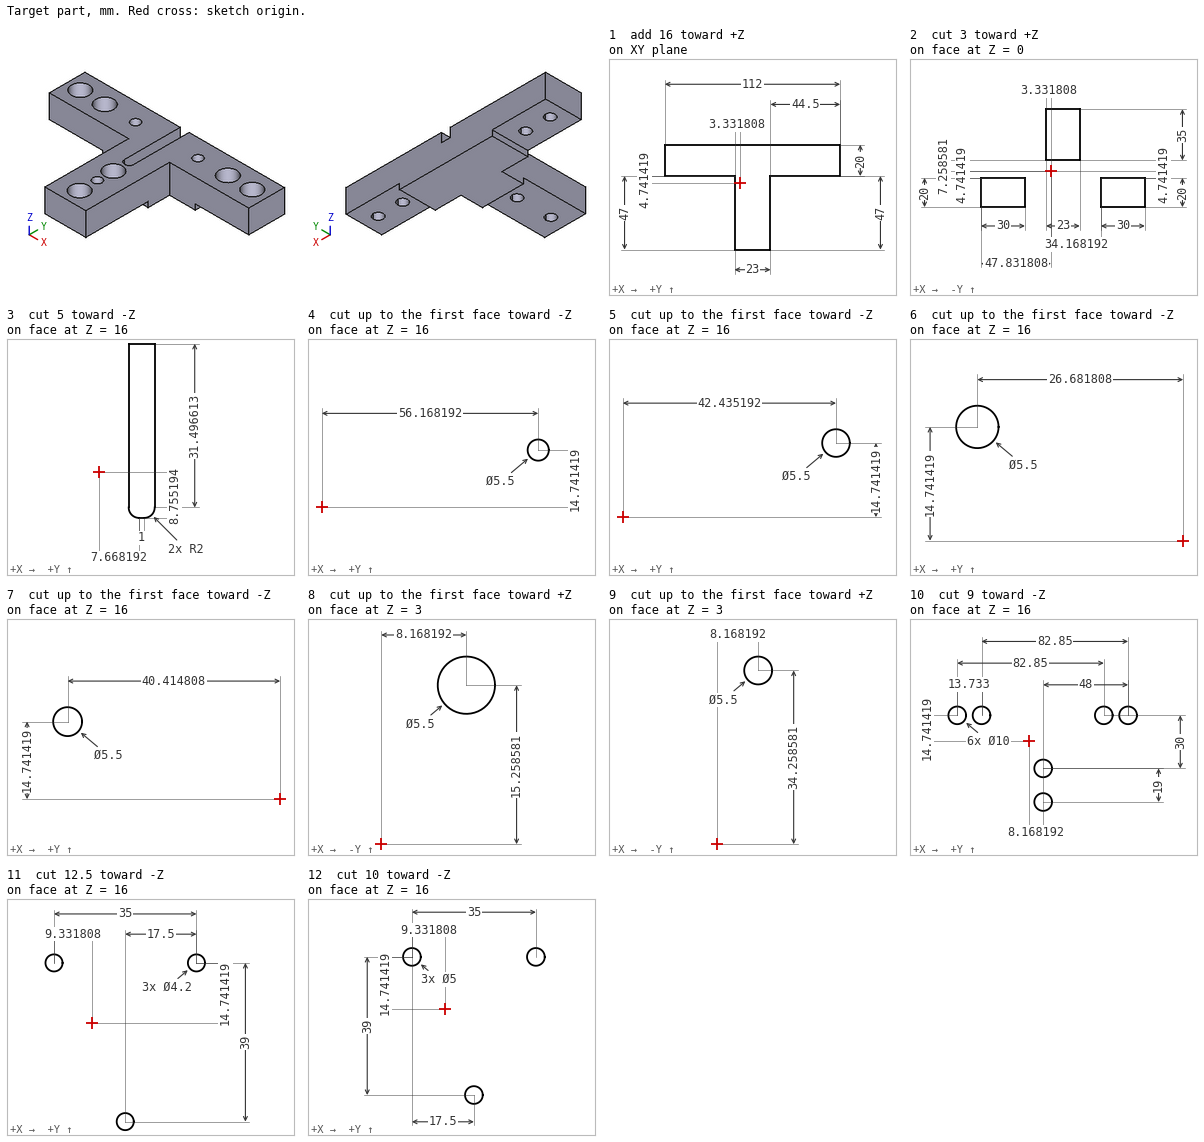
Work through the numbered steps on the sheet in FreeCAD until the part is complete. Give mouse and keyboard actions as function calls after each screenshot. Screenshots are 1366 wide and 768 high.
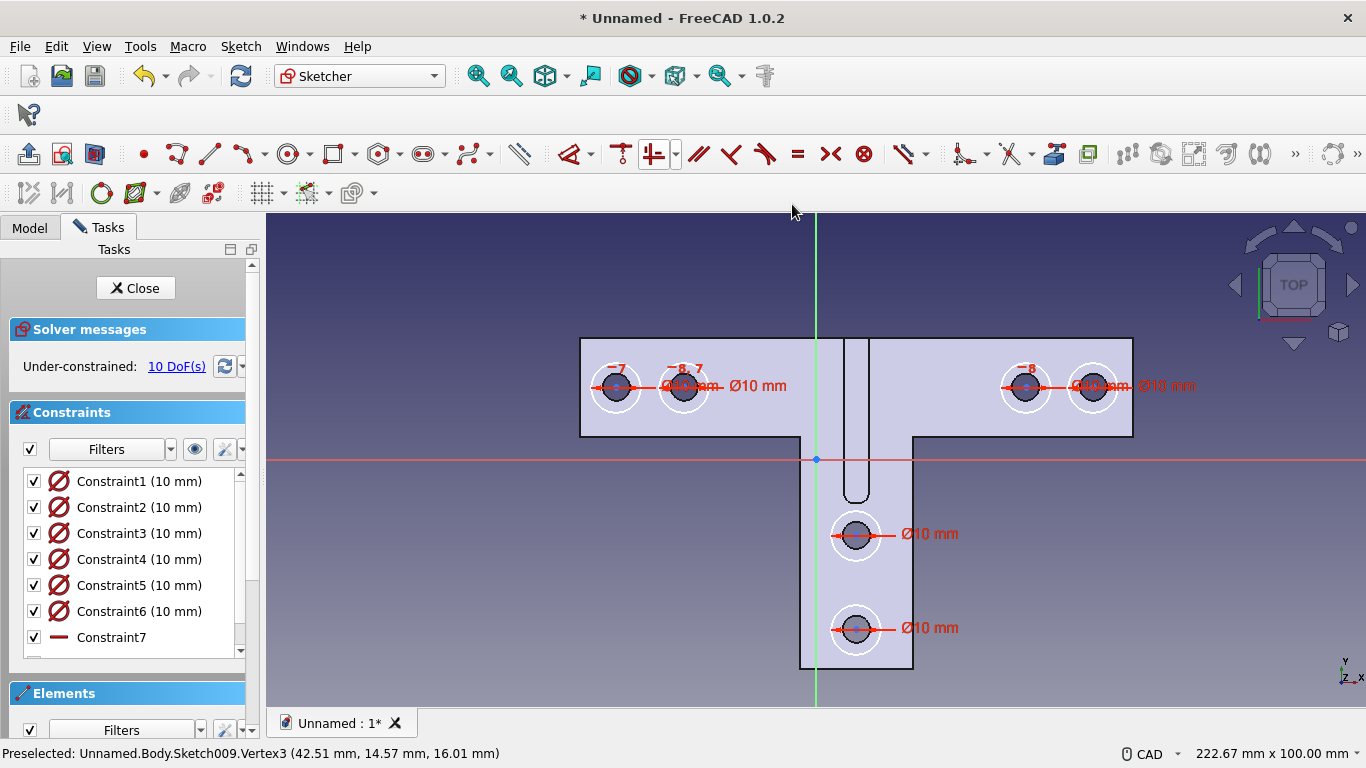
click(1026, 388)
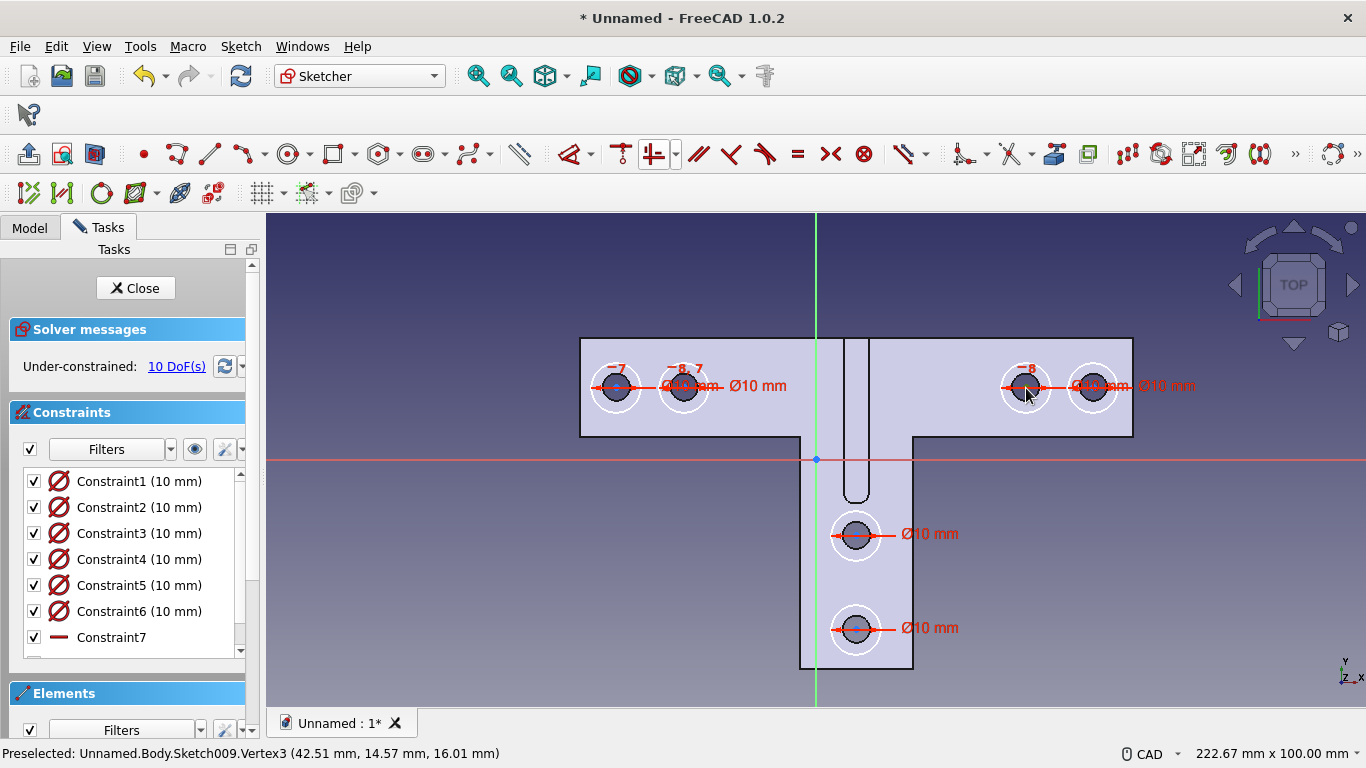
click(1093, 388)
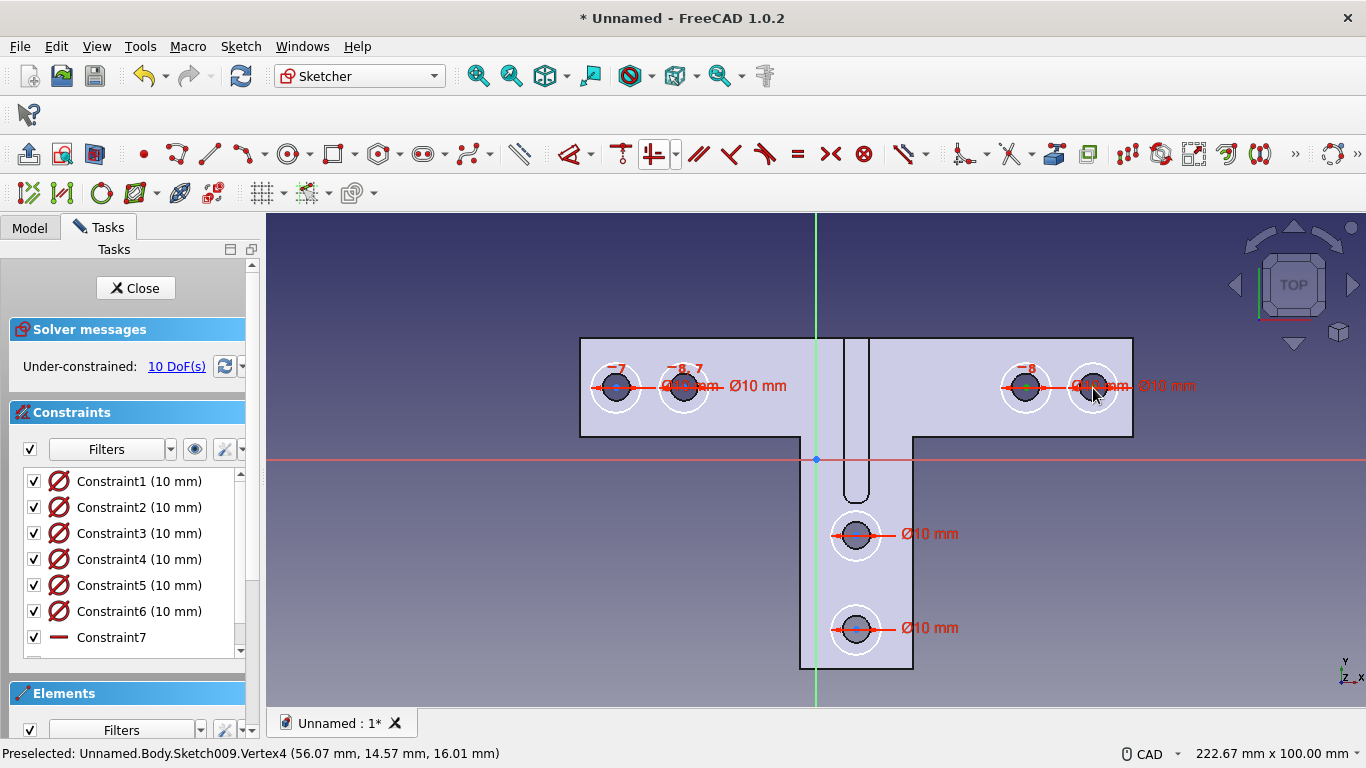
click(676, 154)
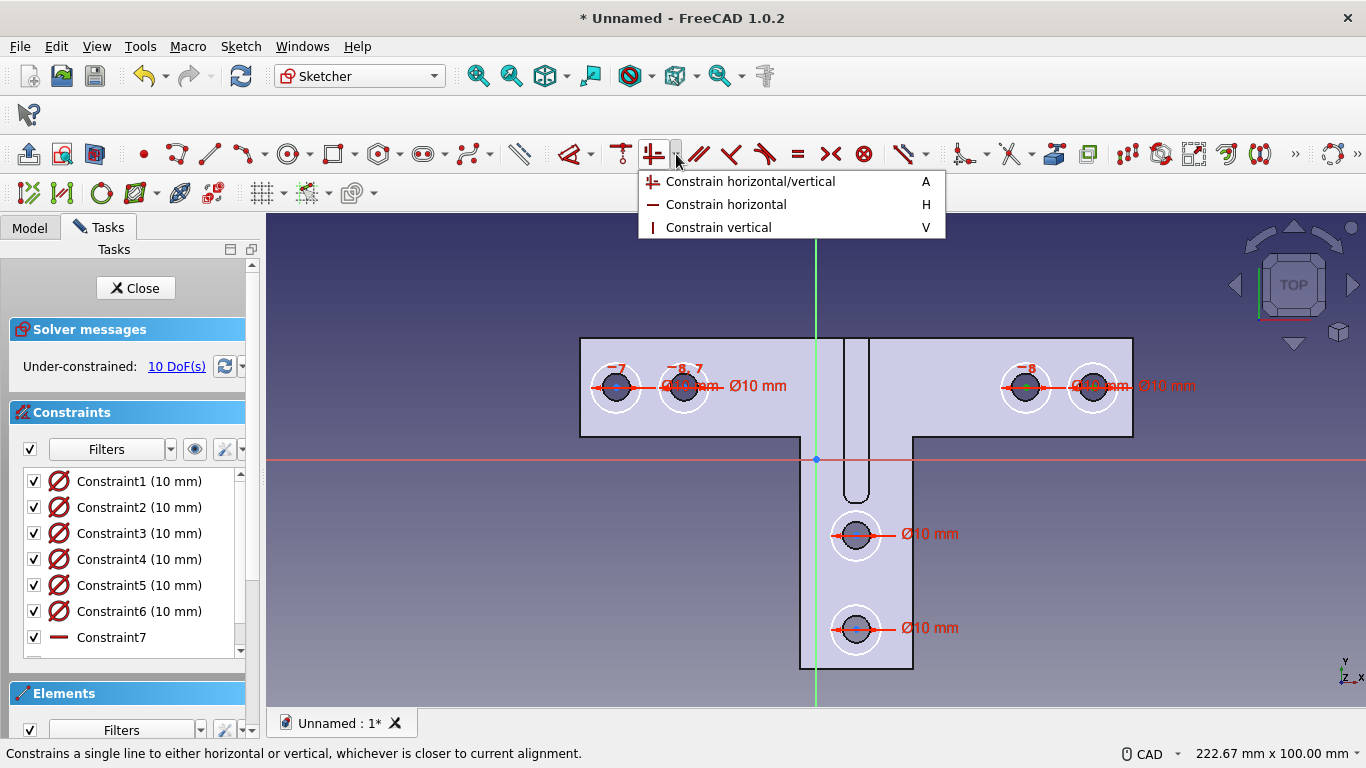
click(792, 204)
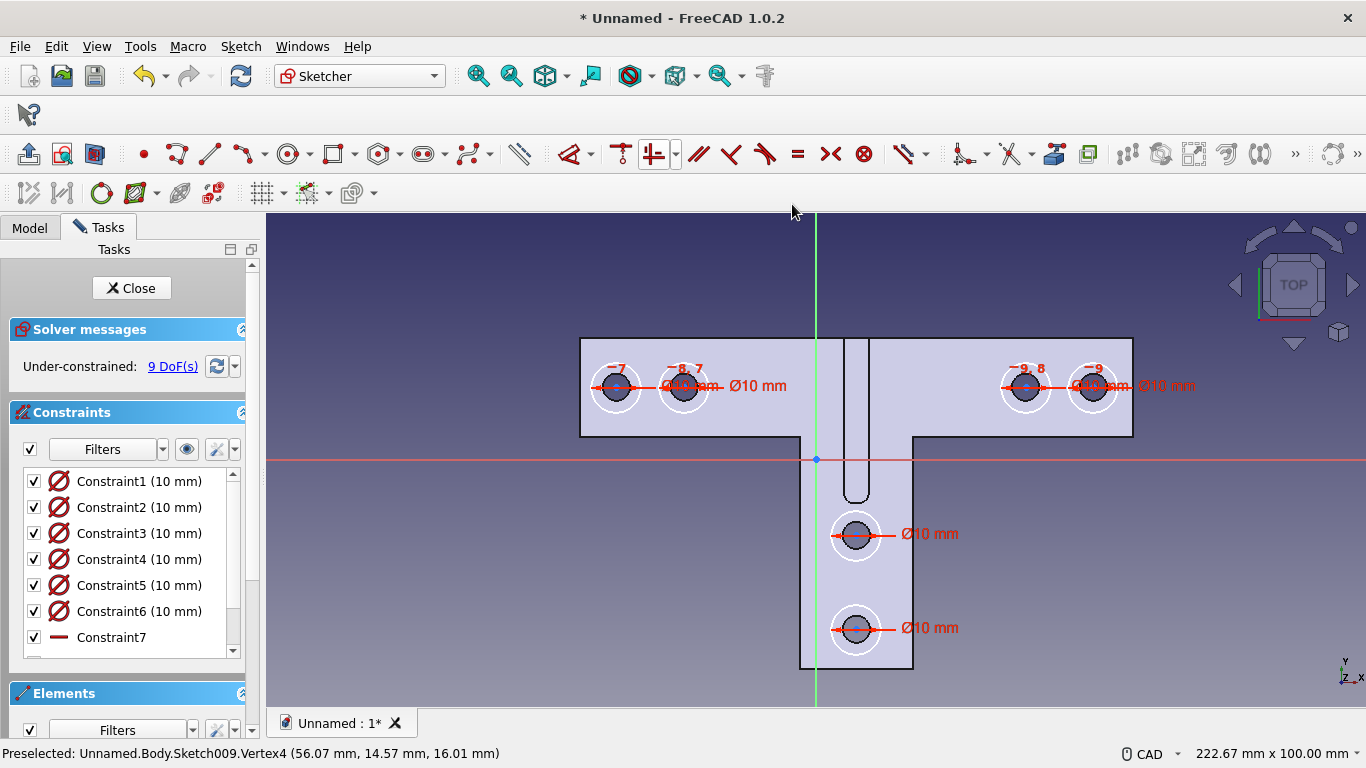
click(856, 536)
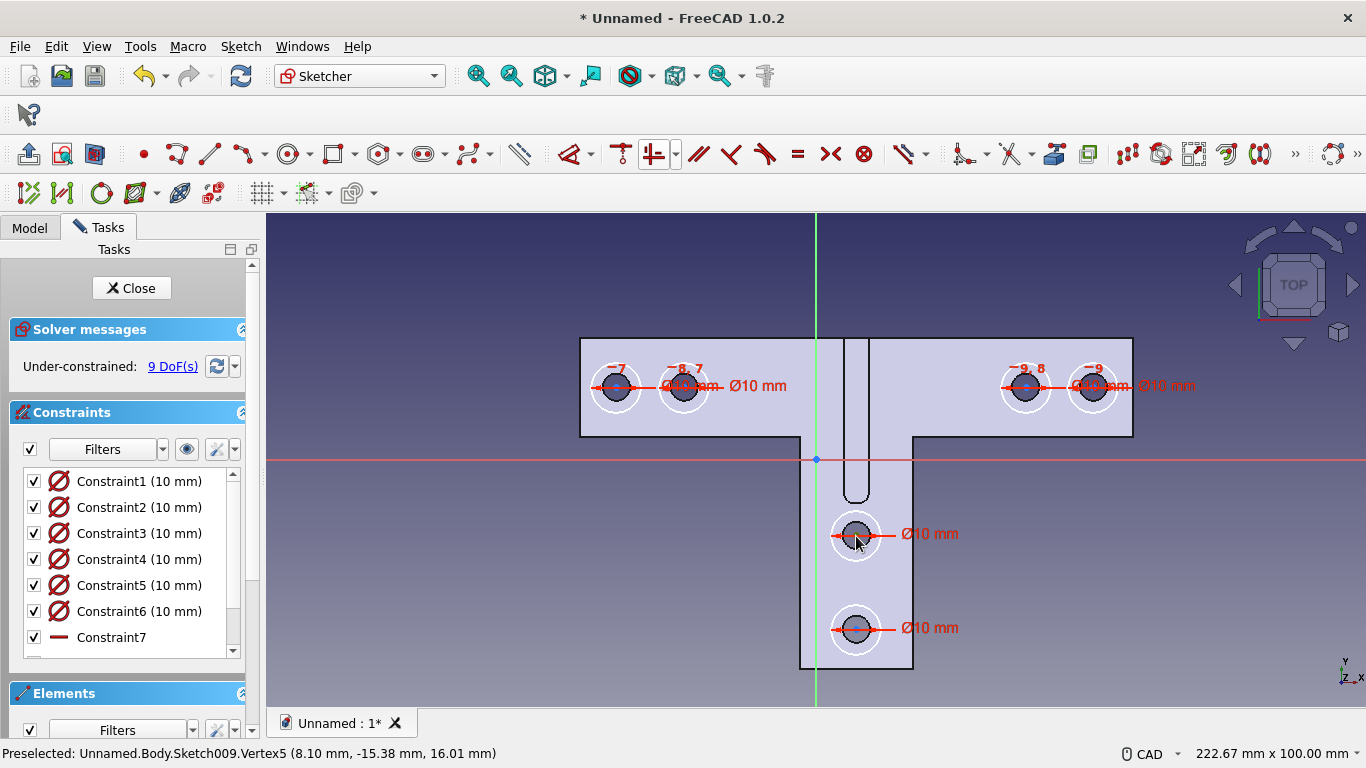
click(856, 630)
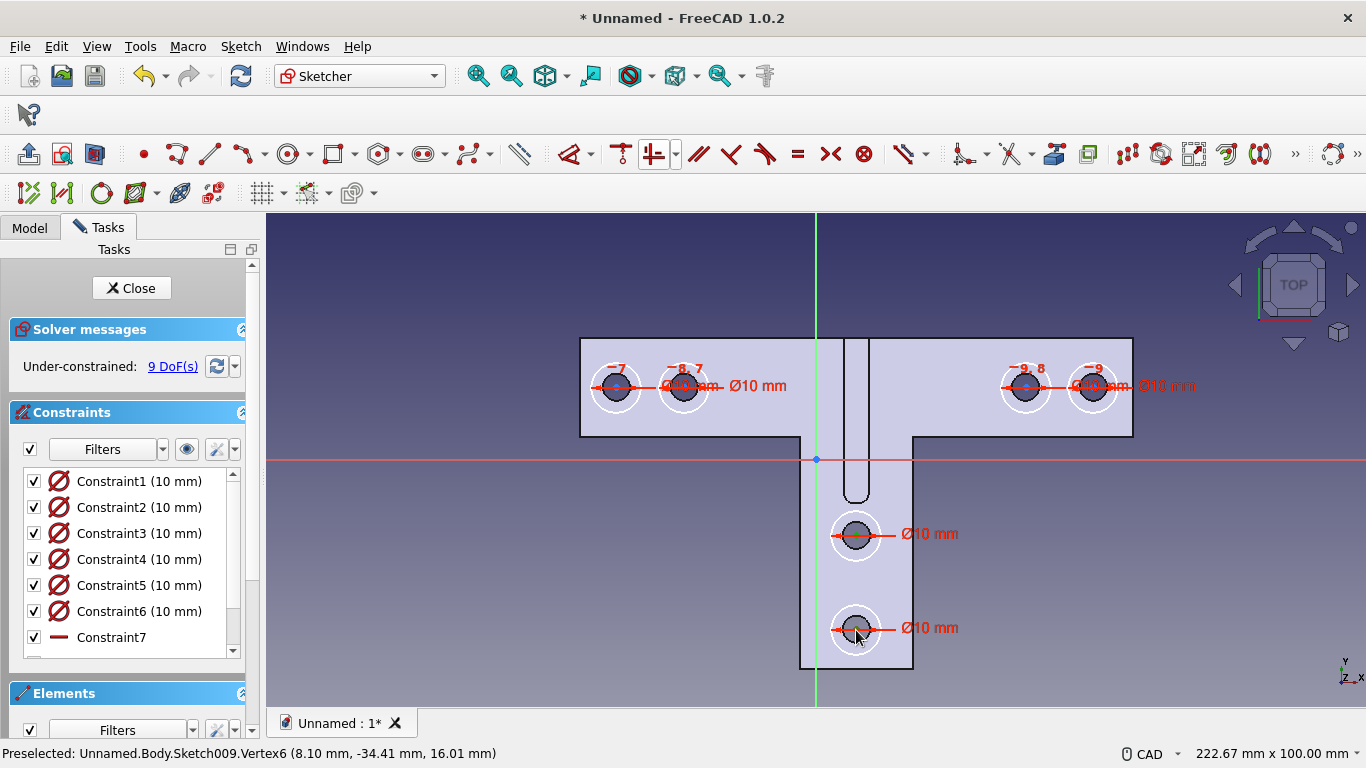
key(v)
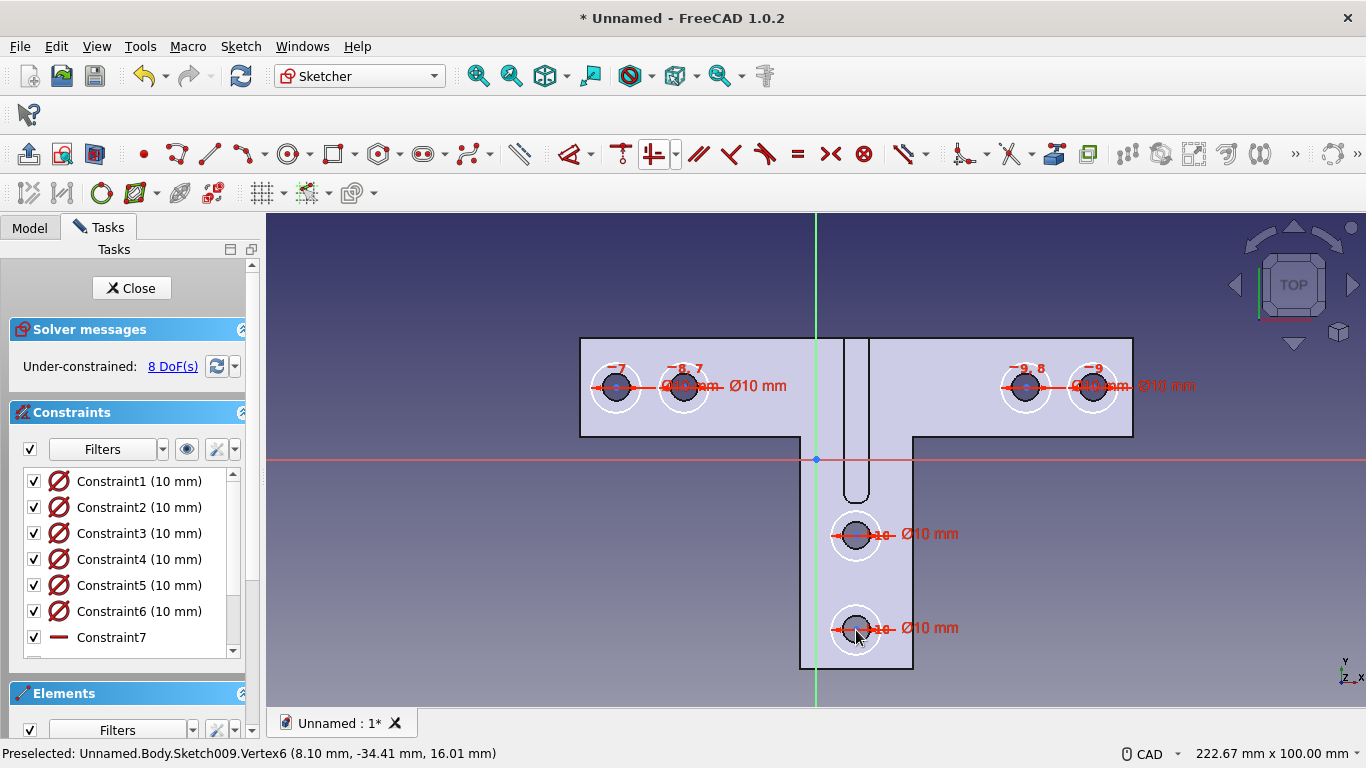
click(568, 154)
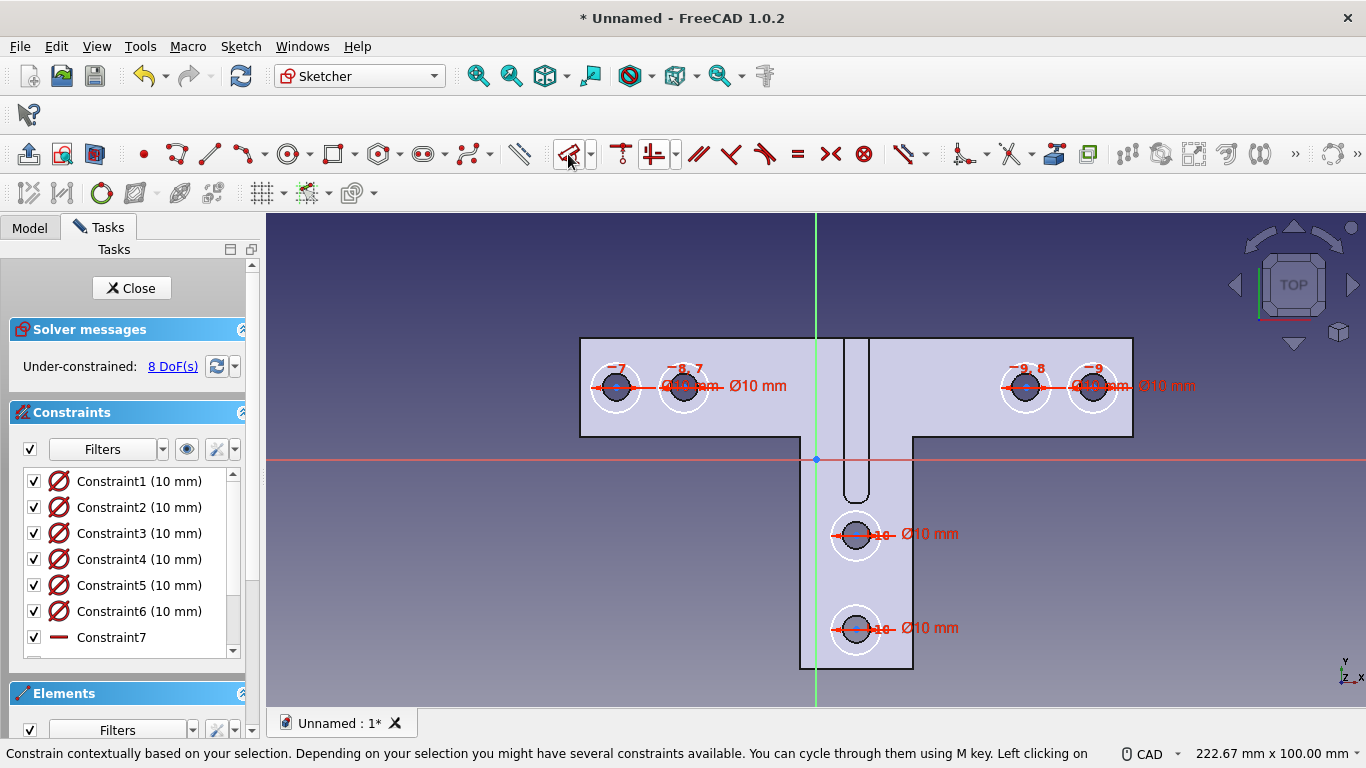
click(1093, 388)